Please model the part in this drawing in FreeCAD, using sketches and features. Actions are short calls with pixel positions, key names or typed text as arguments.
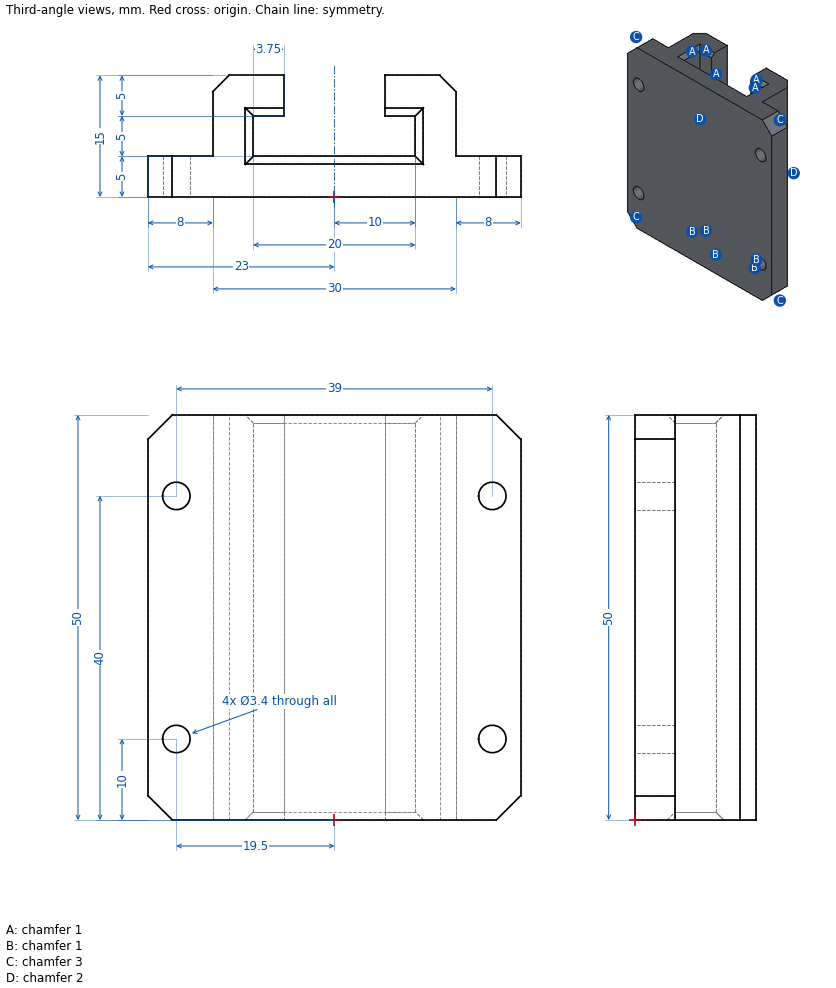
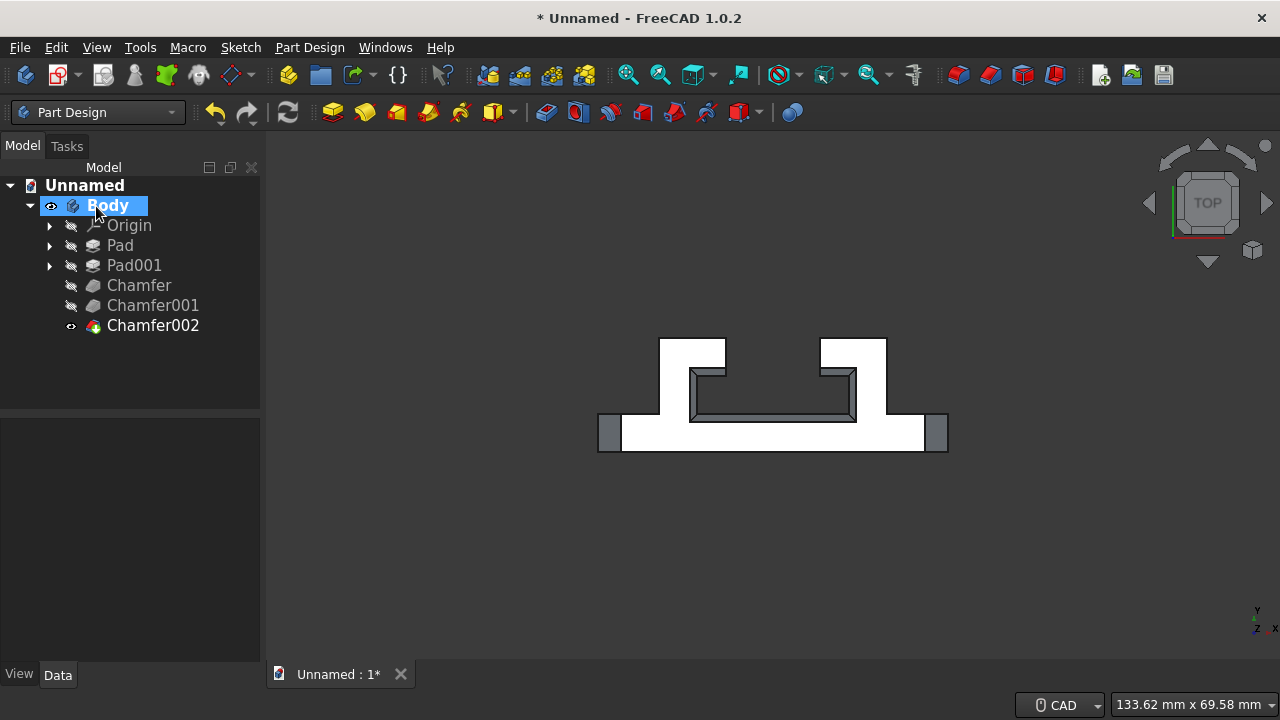
key(4)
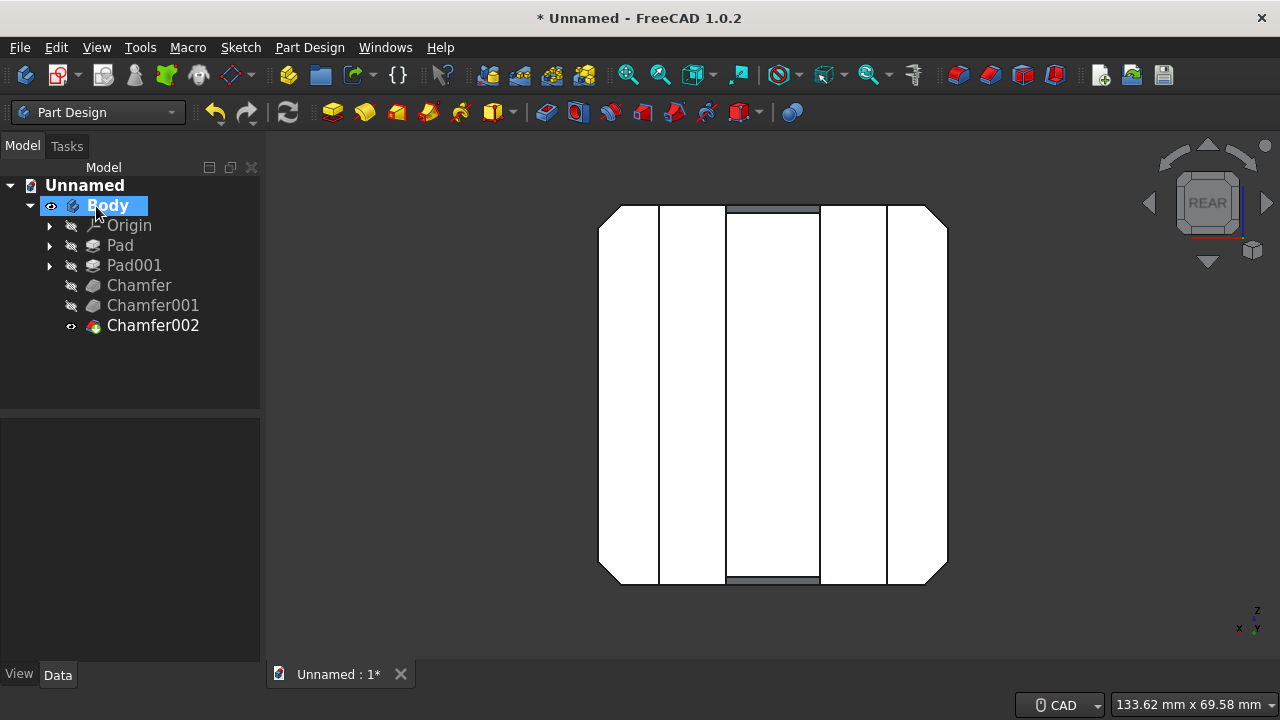
click(773, 290)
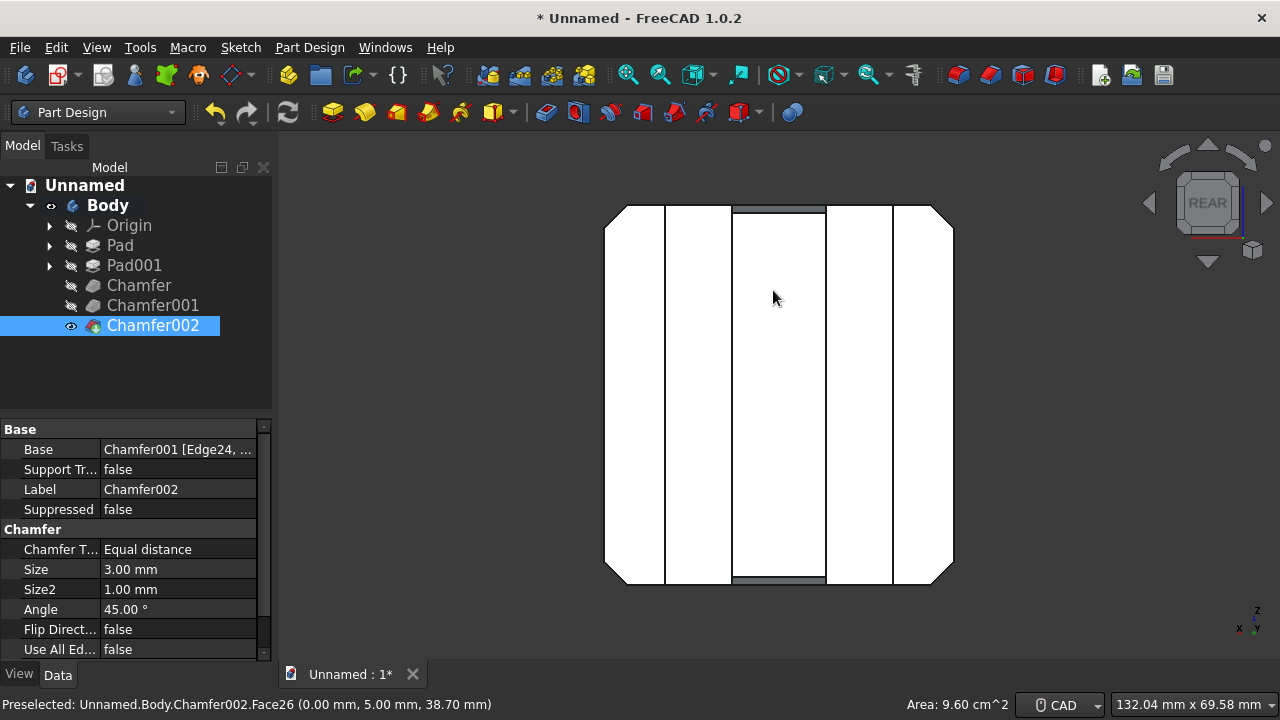
click(58, 76)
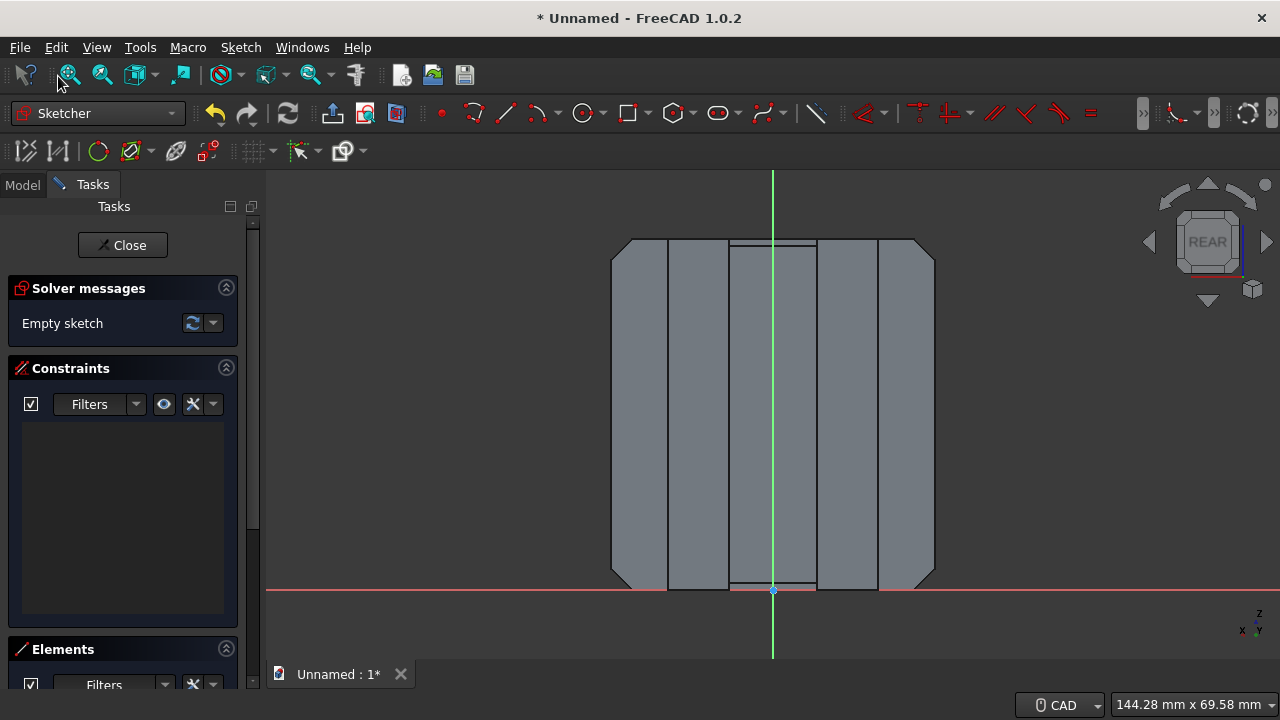
key(q)
key(s)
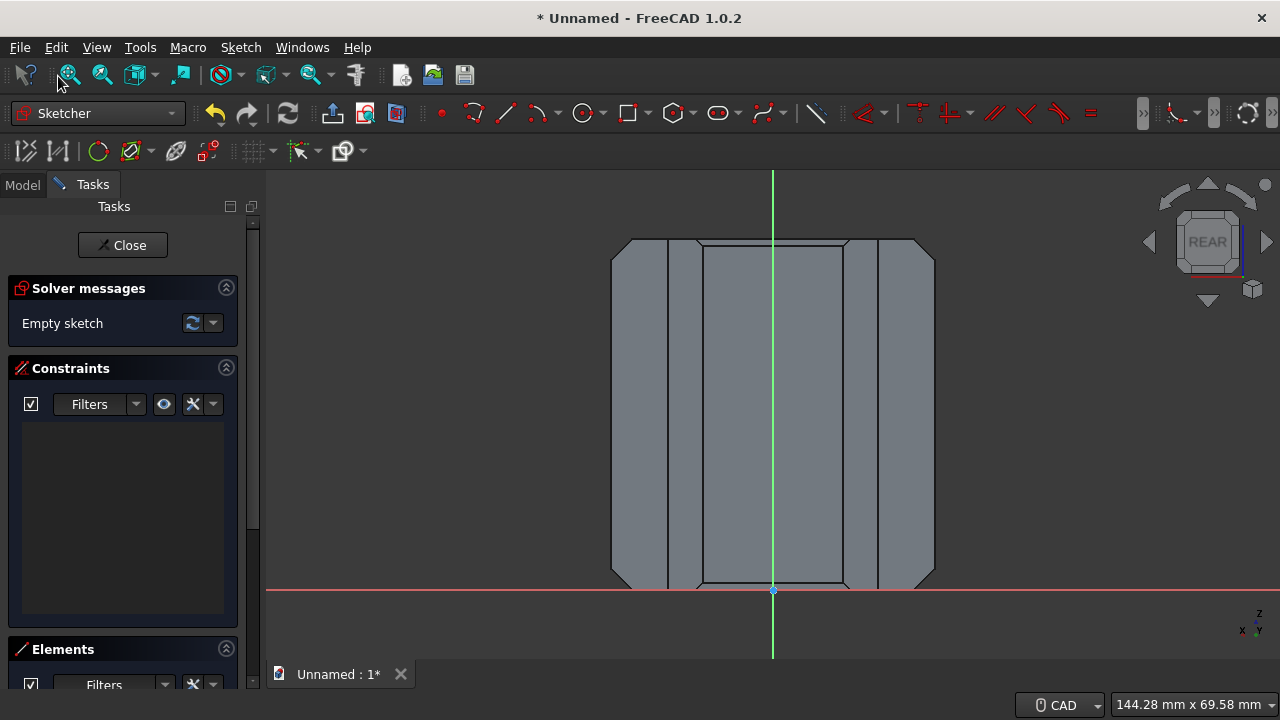
key(g)
key(c)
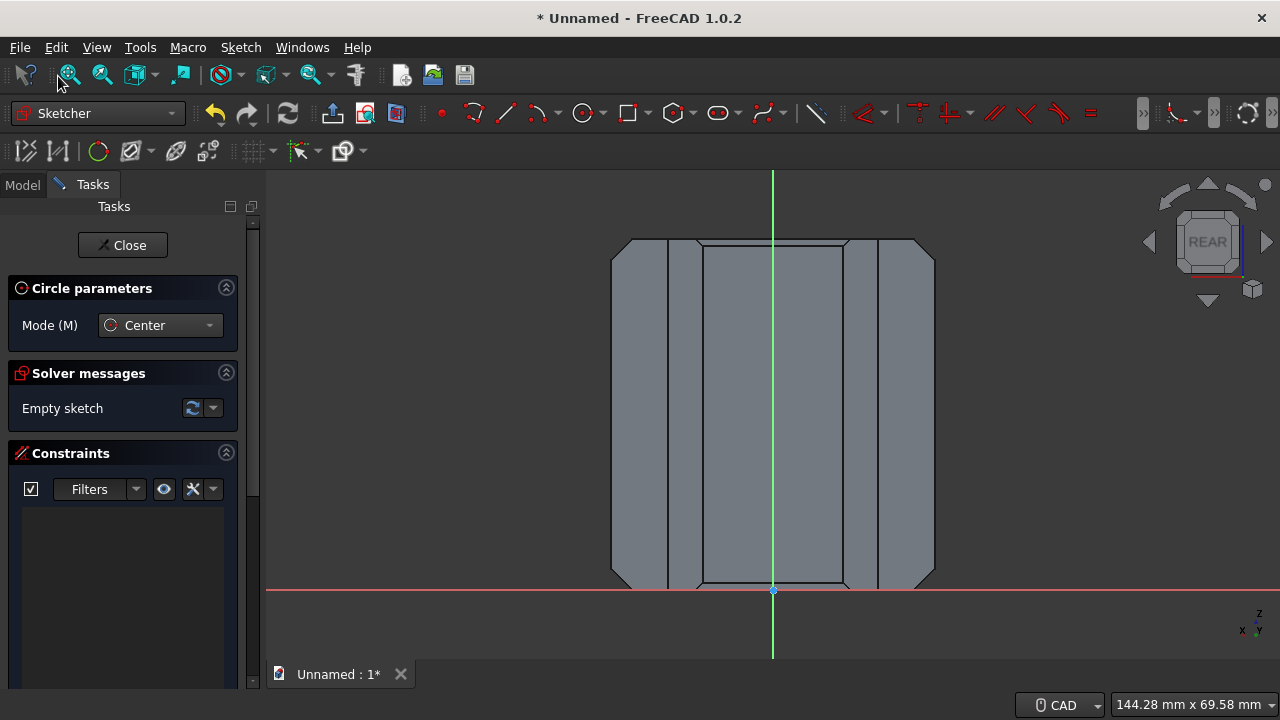
scroll(910, 520, up, 4)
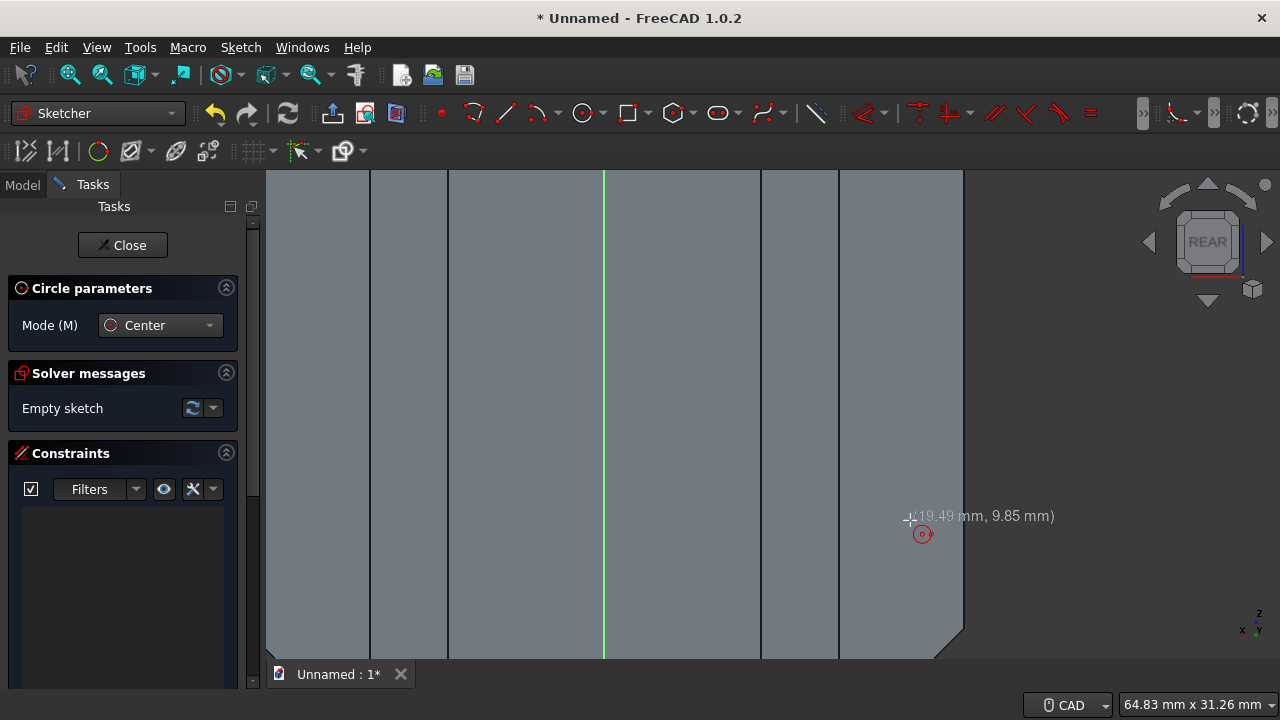
click(909, 519)
click(928, 500)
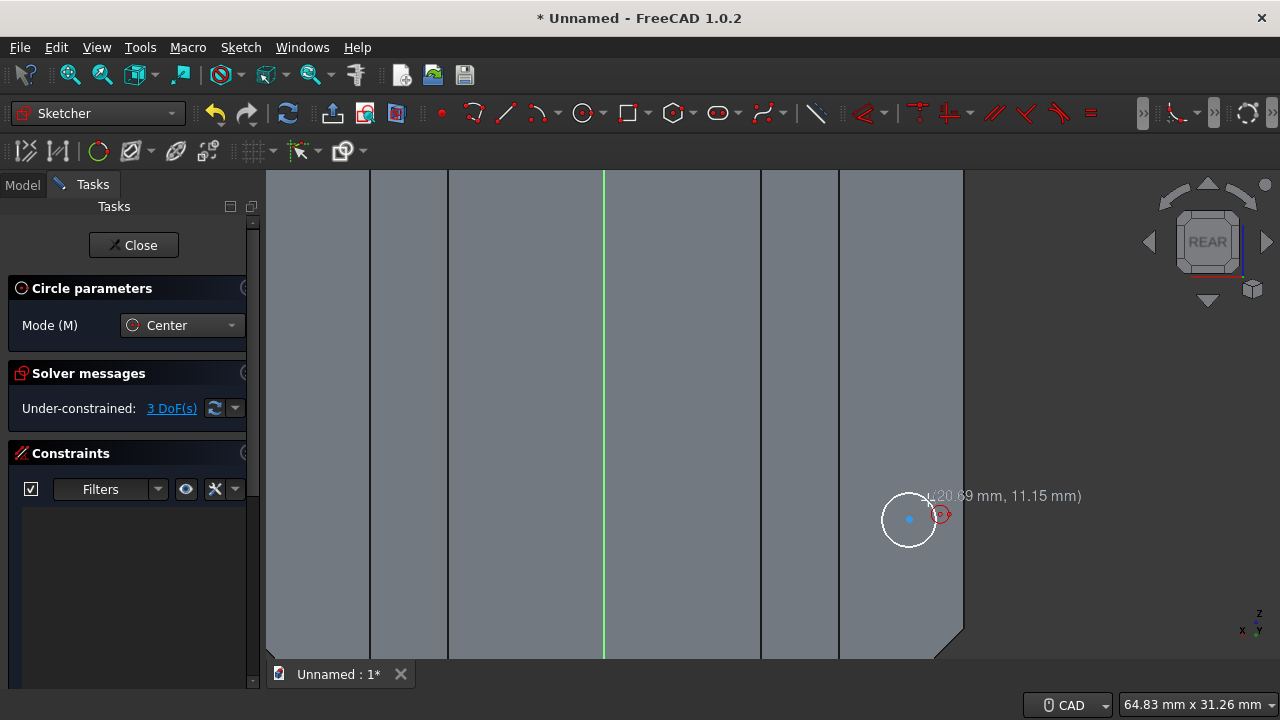
scroll(786, 468, down, 4)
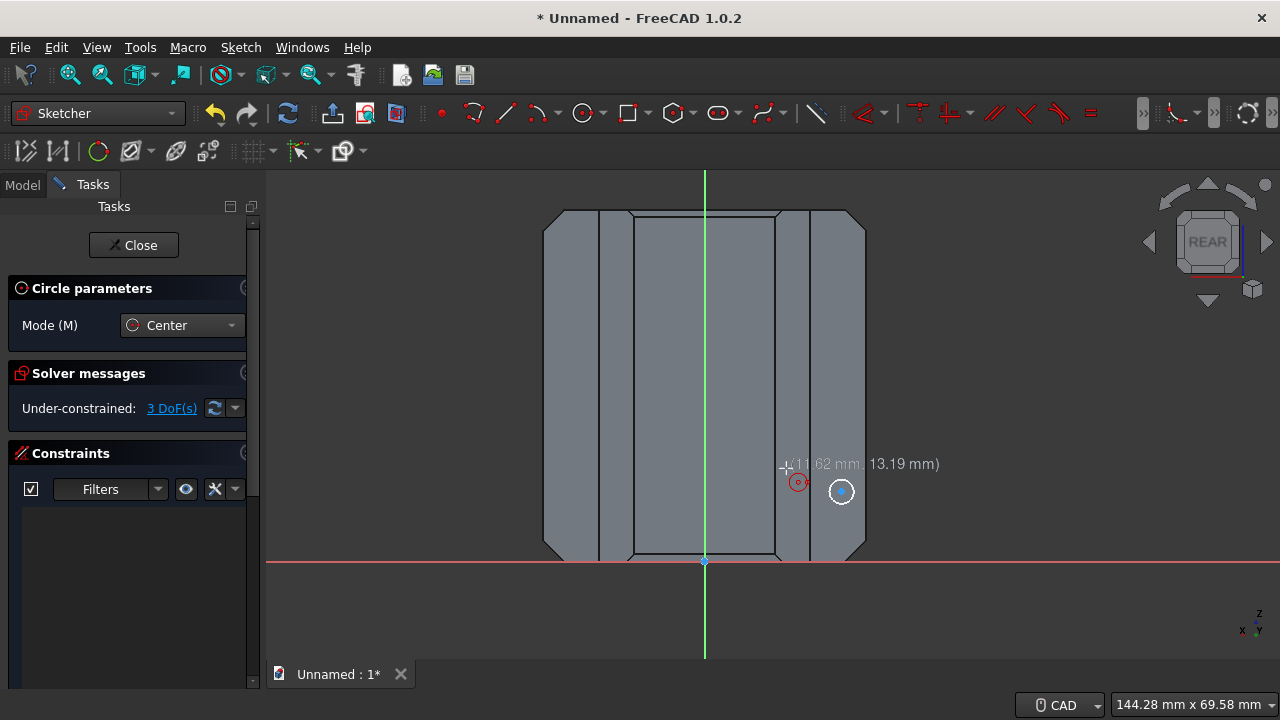
scroll(842, 280, up, 4)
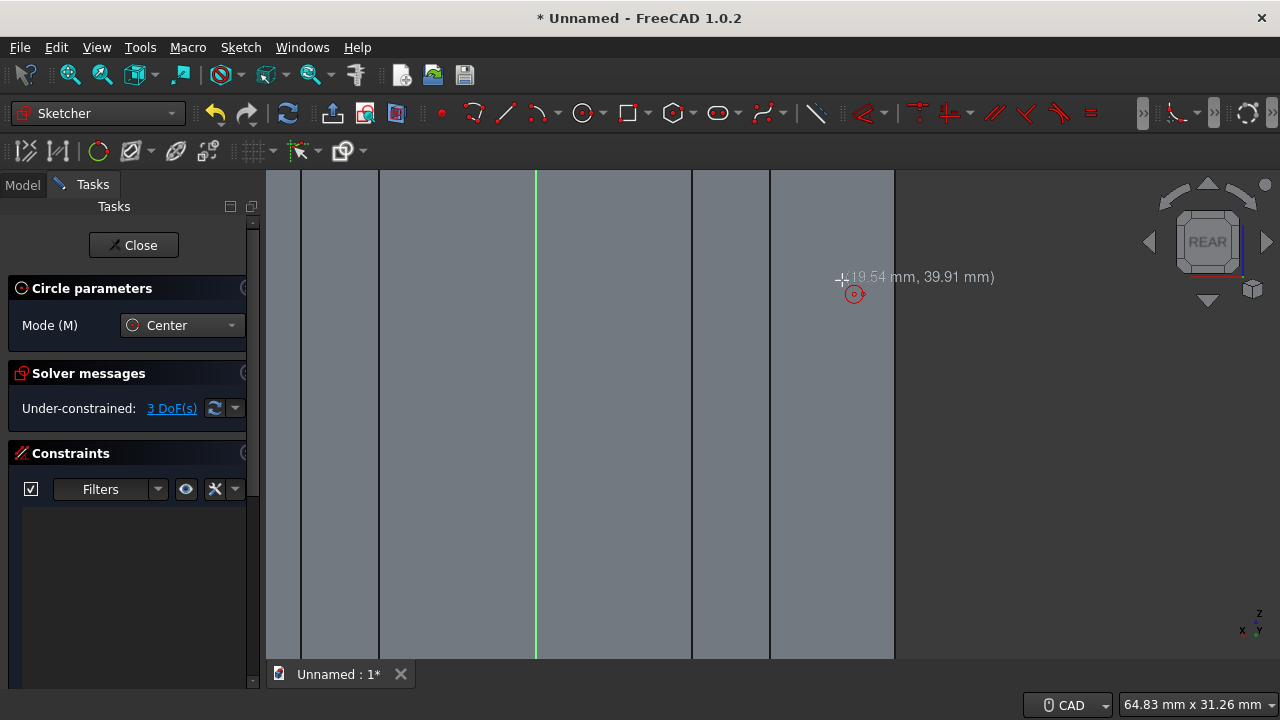
click(841, 281)
click(859, 262)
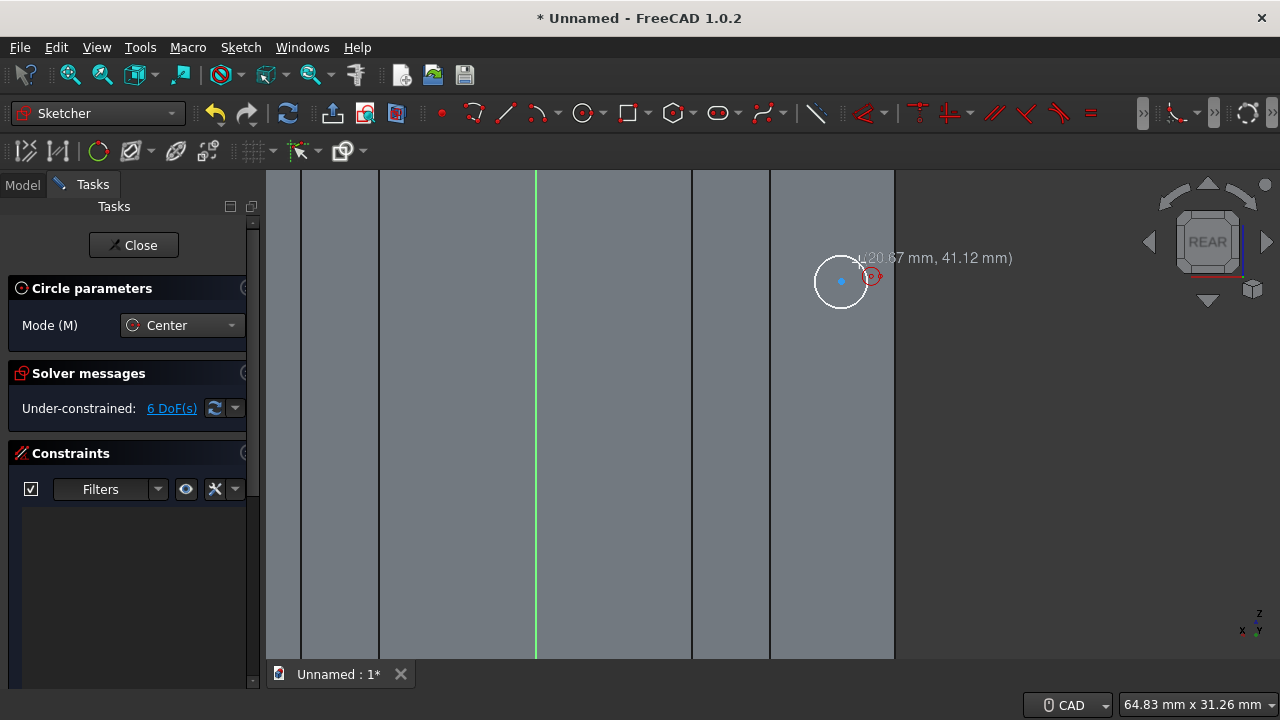
scroll(842, 279, down, 4)